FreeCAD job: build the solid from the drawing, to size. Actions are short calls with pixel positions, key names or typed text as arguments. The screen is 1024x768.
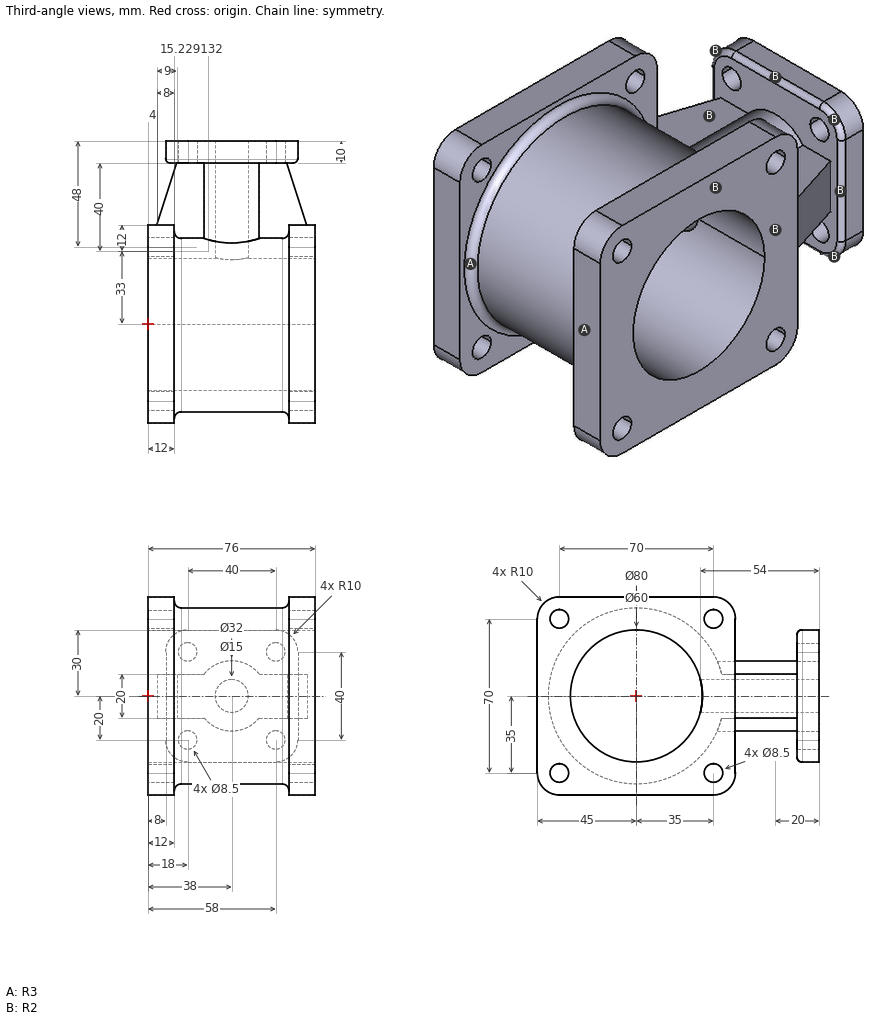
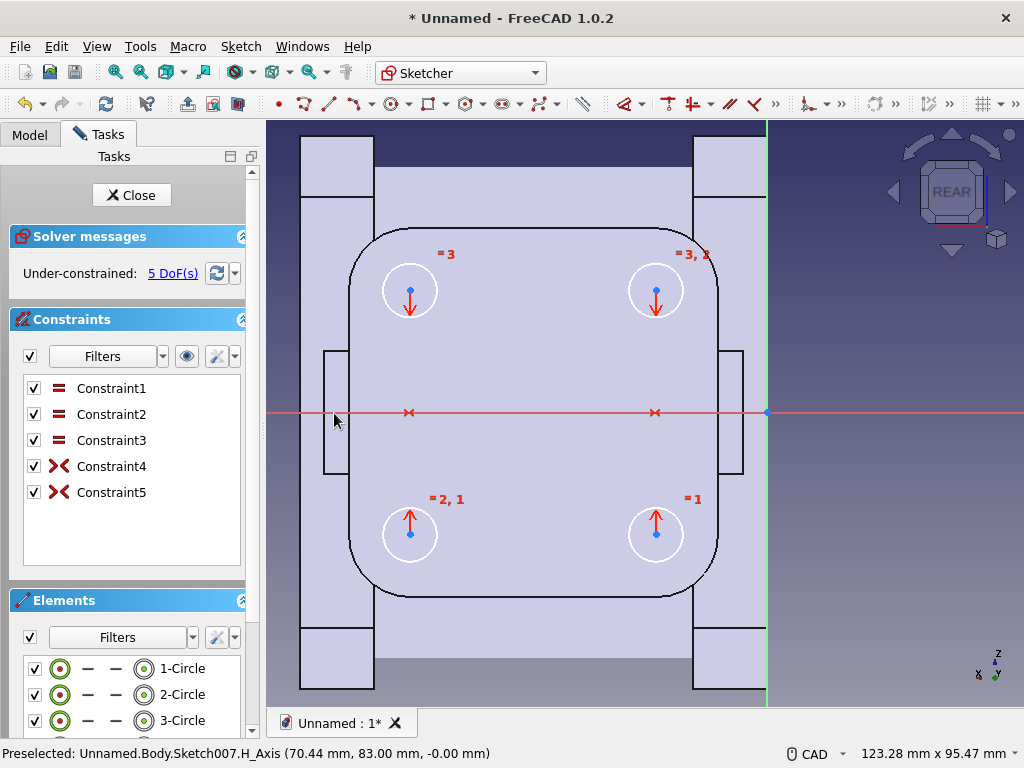
click(675, 516)
click(698, 493)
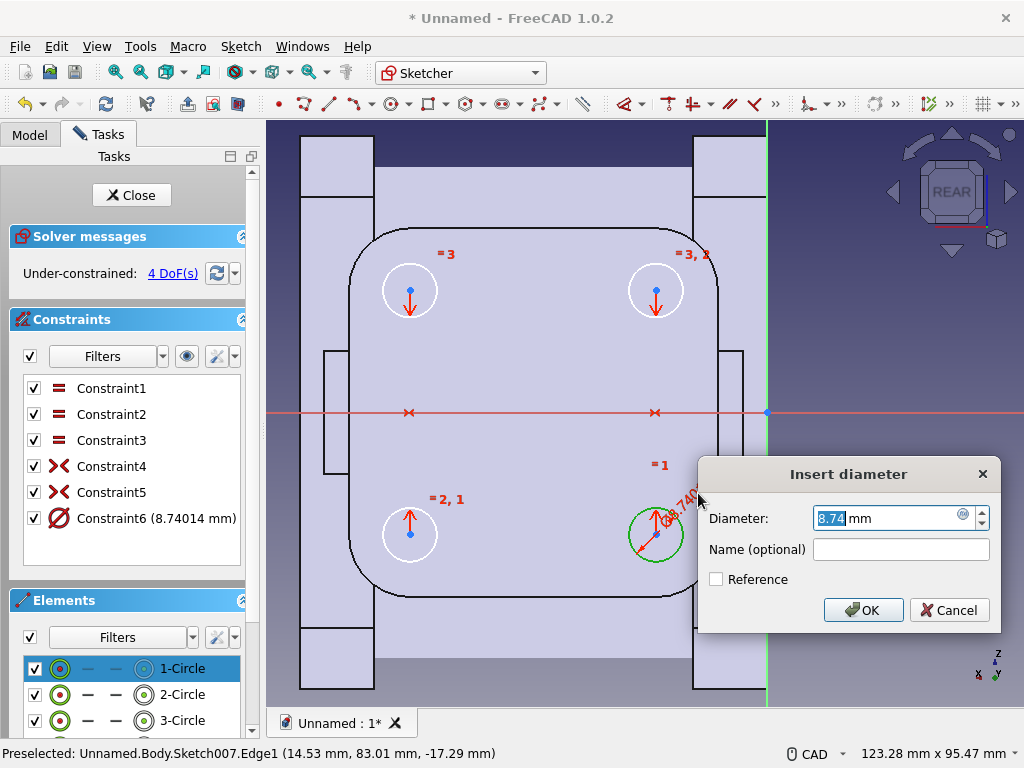
text(8.5)
key(Return)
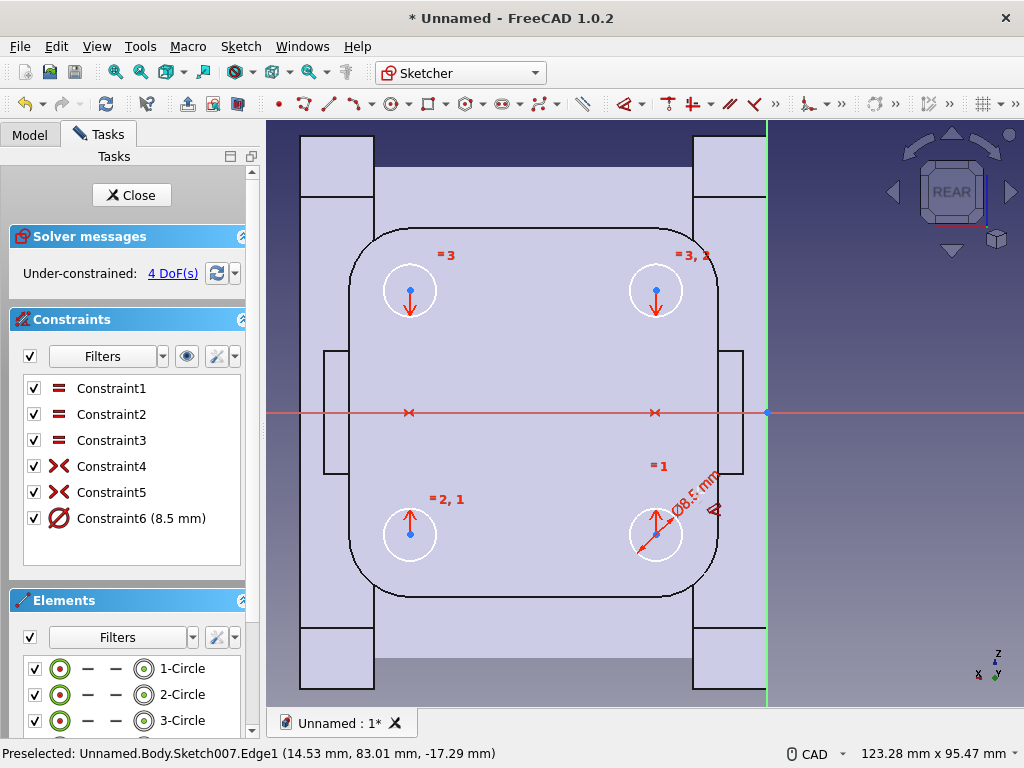
click(656, 535)
click(712, 569)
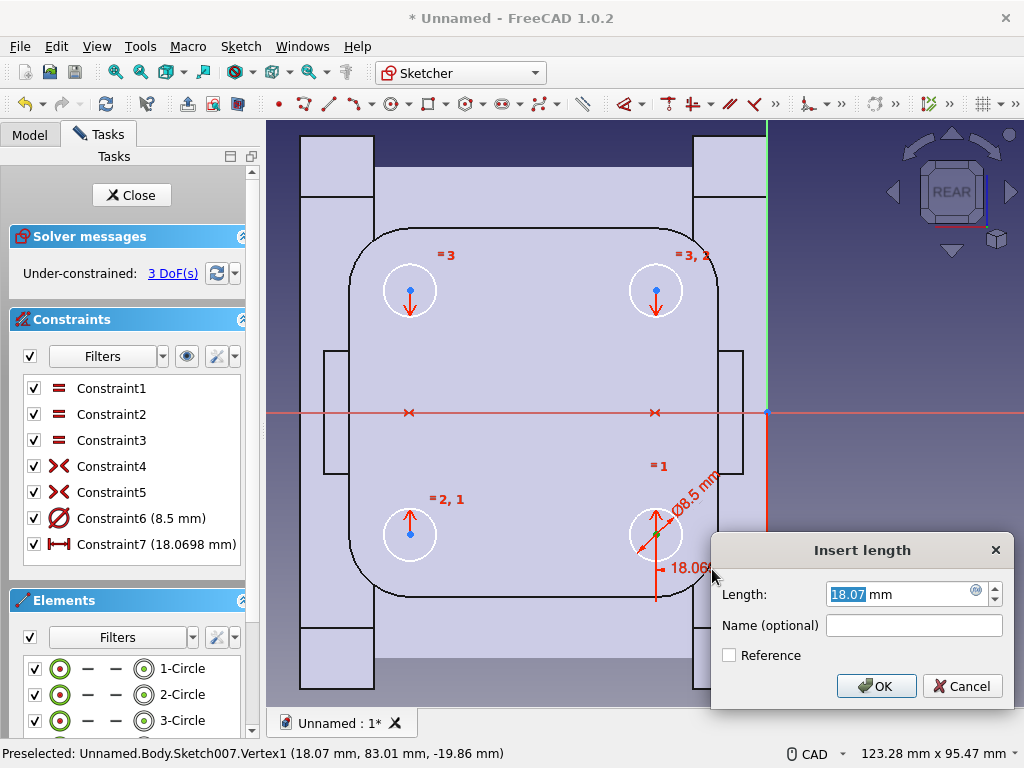
text(18)
key(Return)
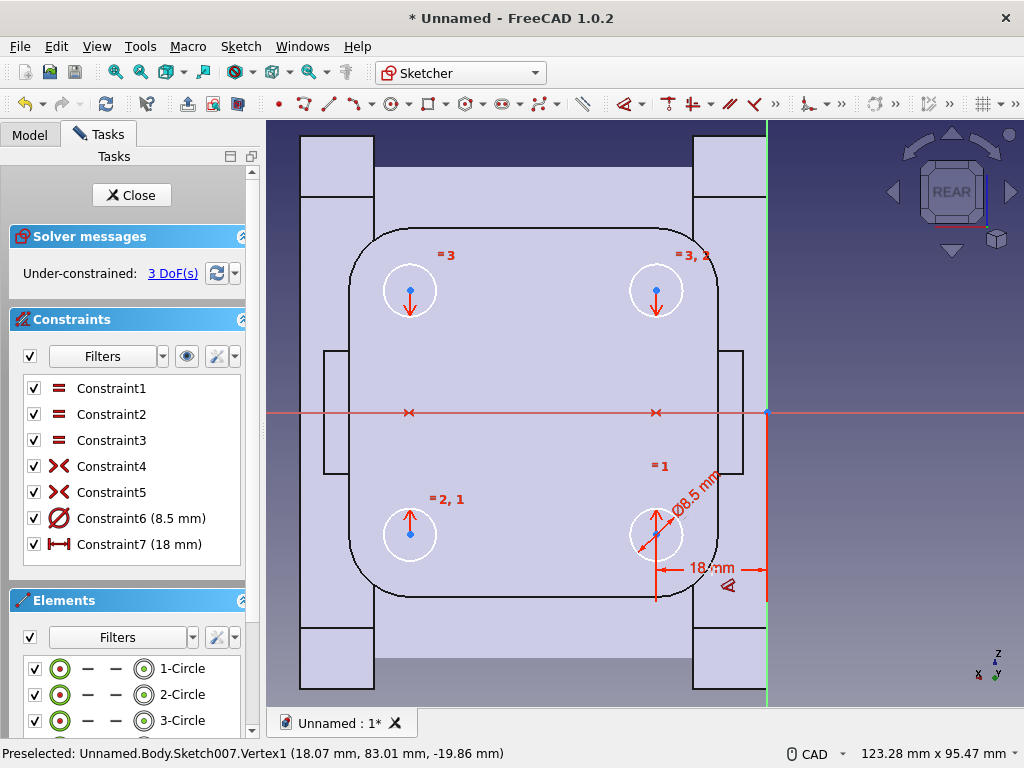
click(656, 535)
click(801, 474)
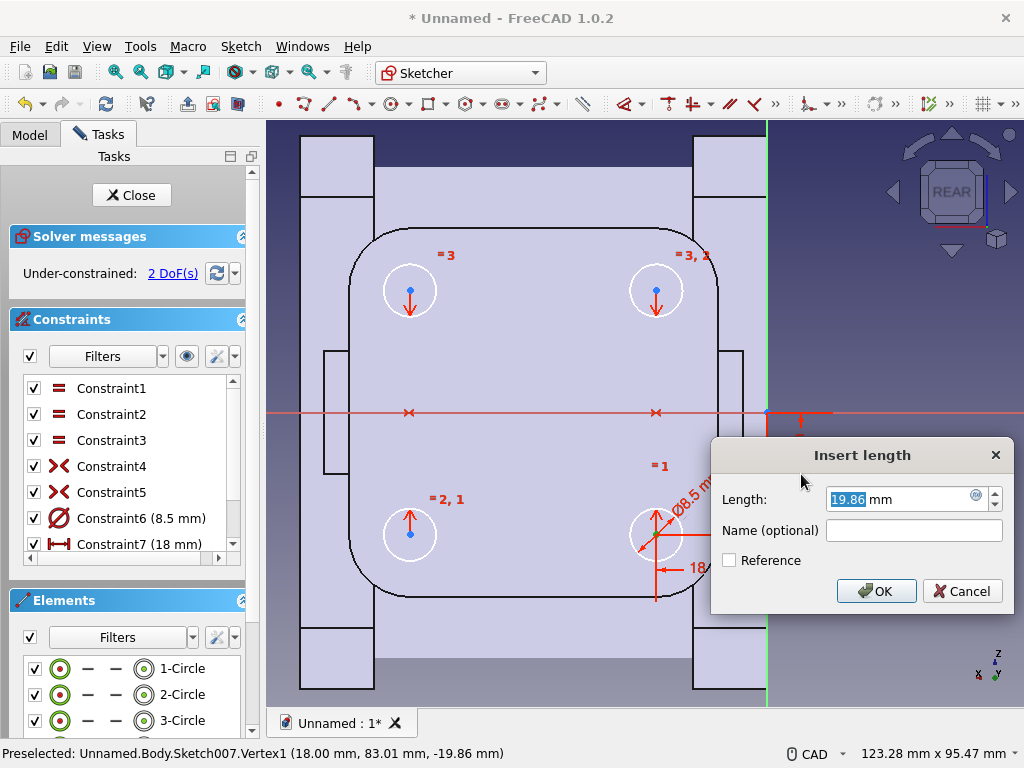
text(20)
key(Return)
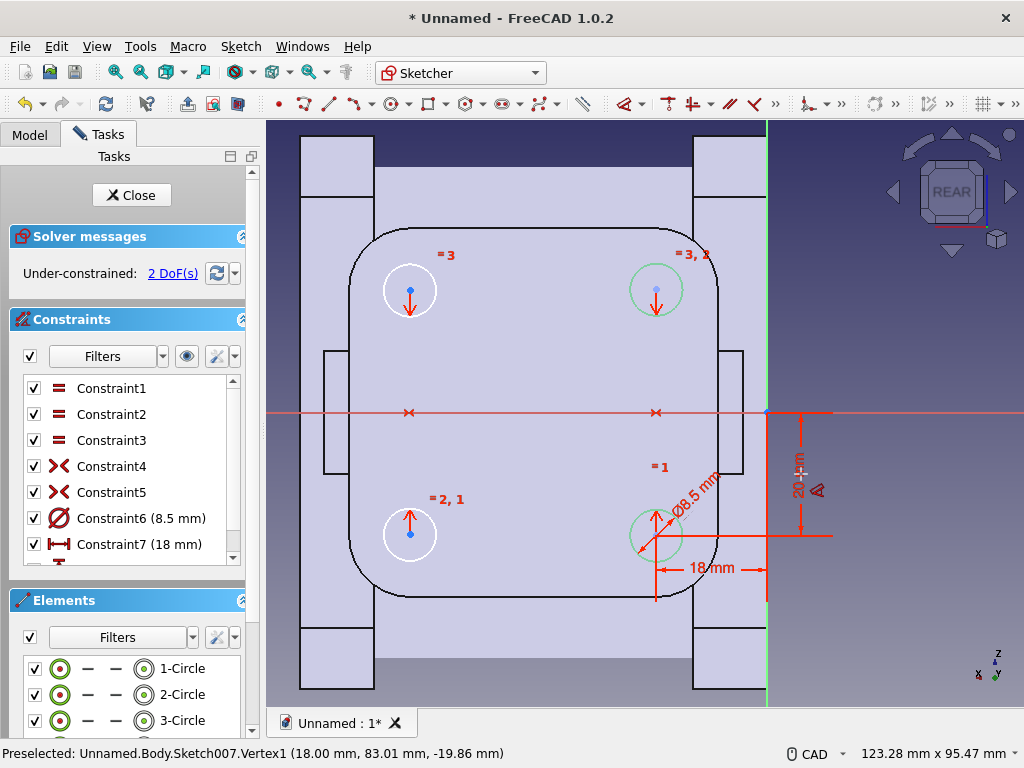
click(410, 535)
click(589, 569)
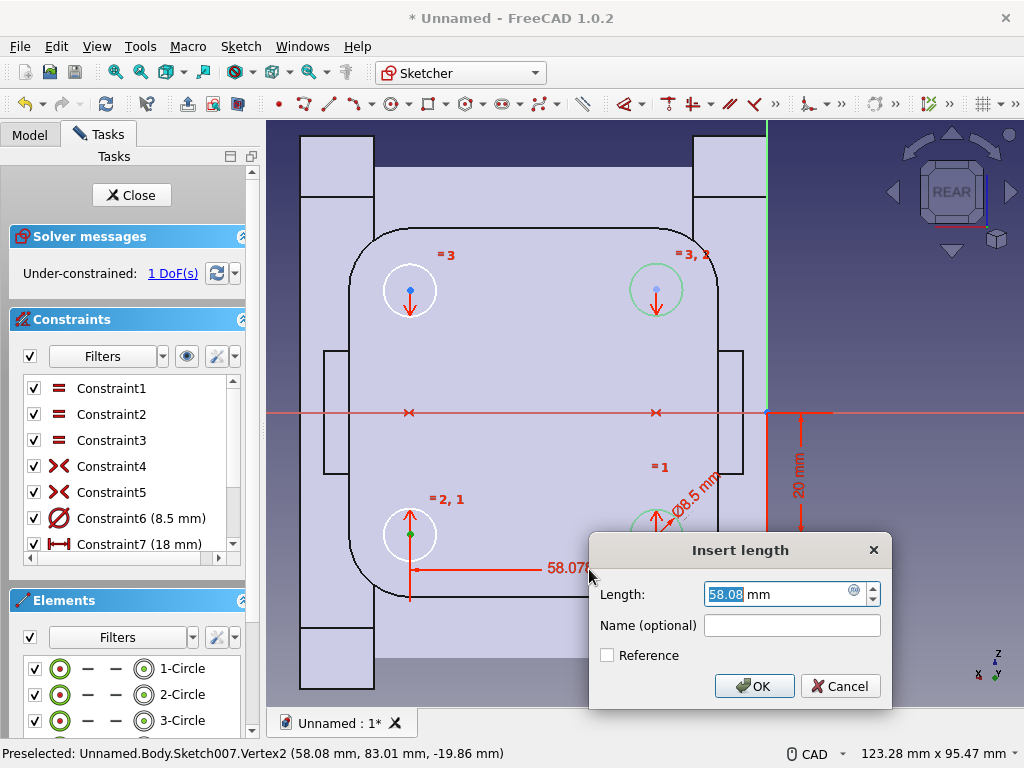
text(58)
key(Return)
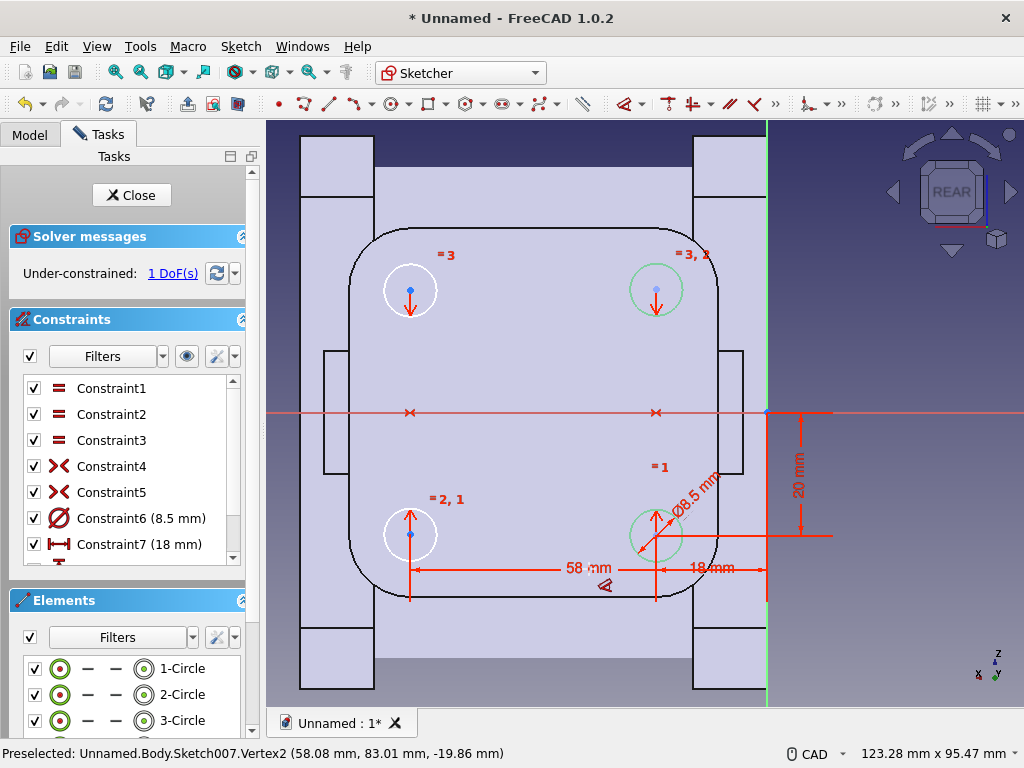
click(410, 535)
click(801, 446)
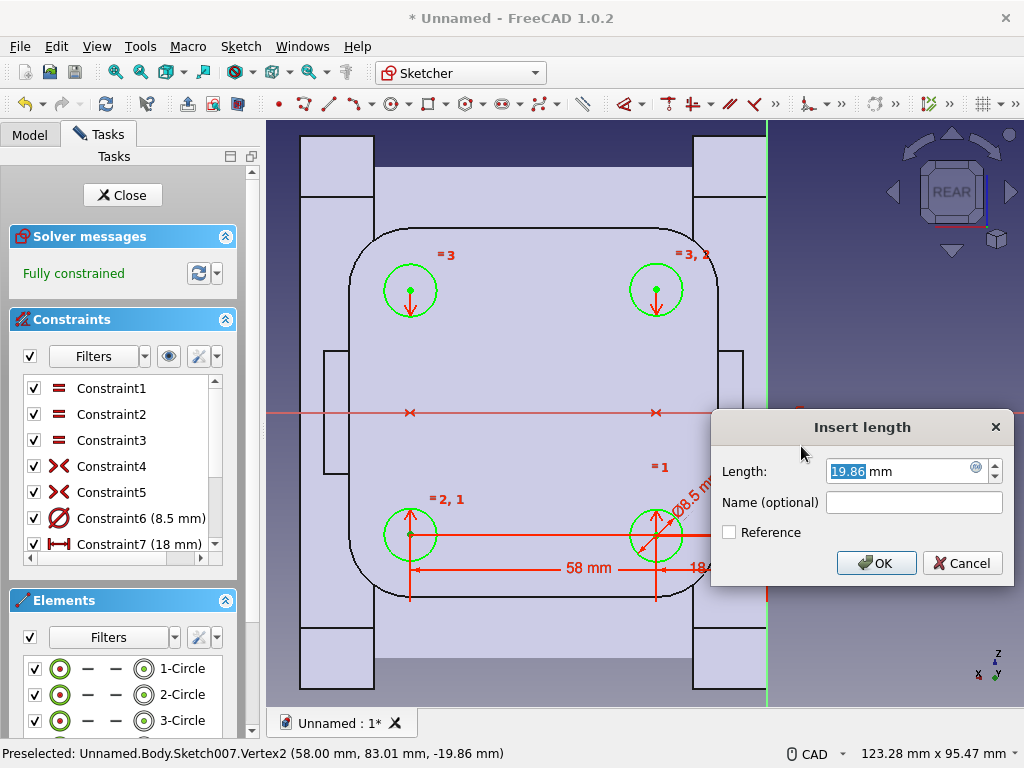
text(20)
key(Return)
key(Escape)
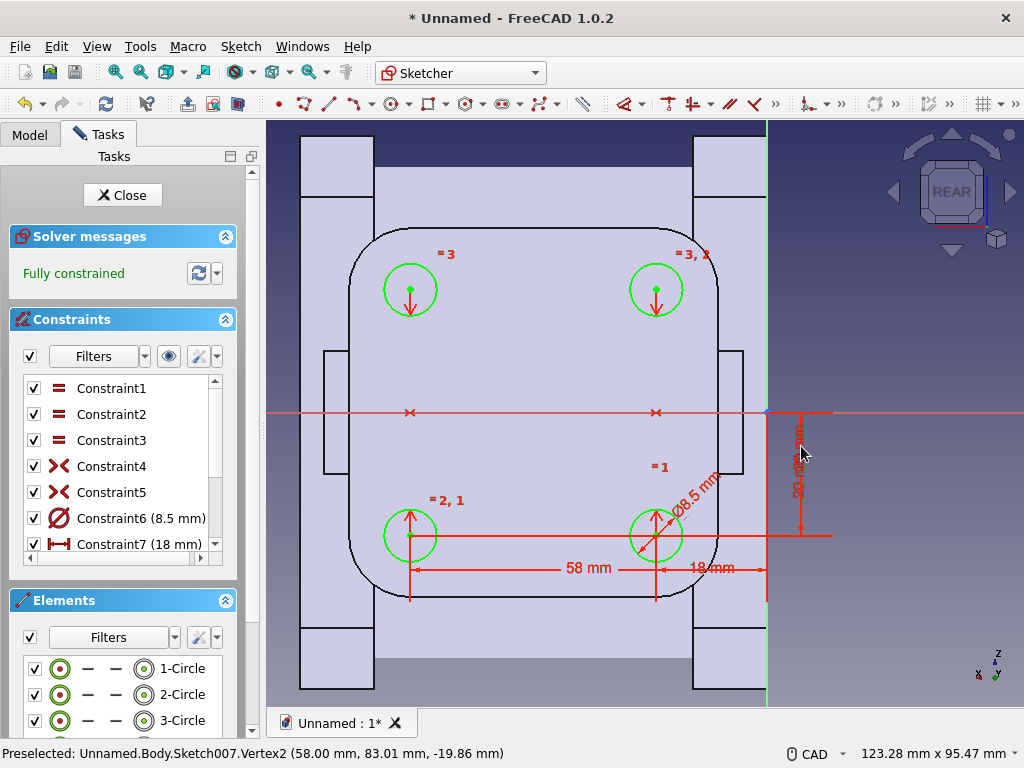
click(123, 195)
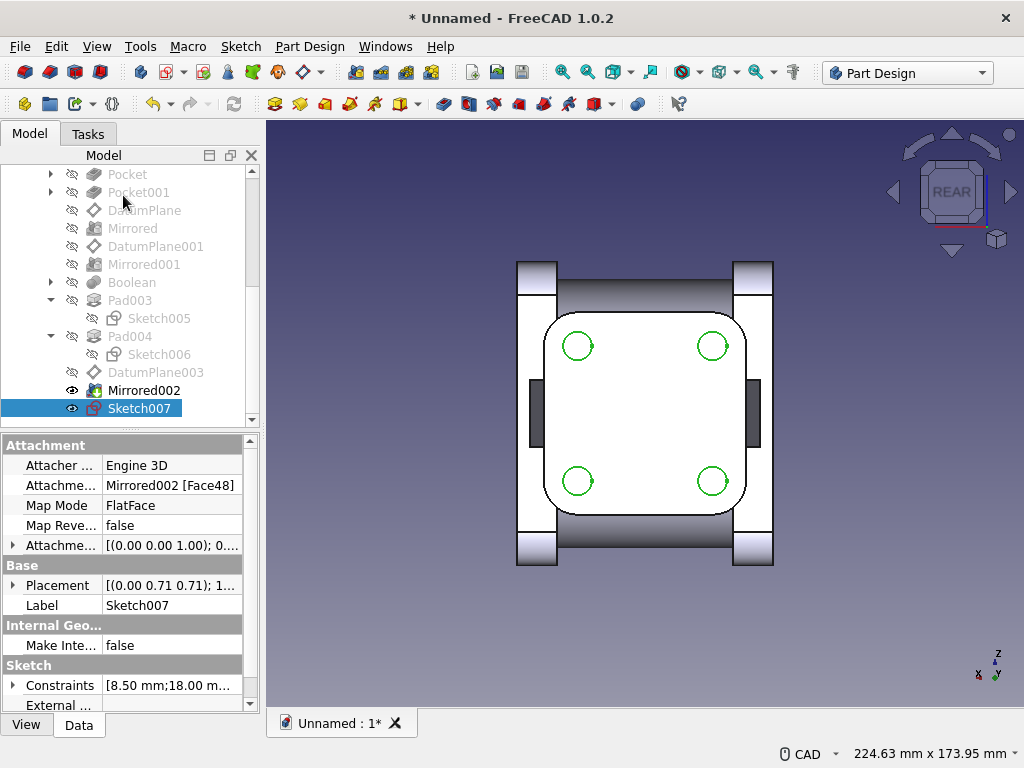
click(444, 104)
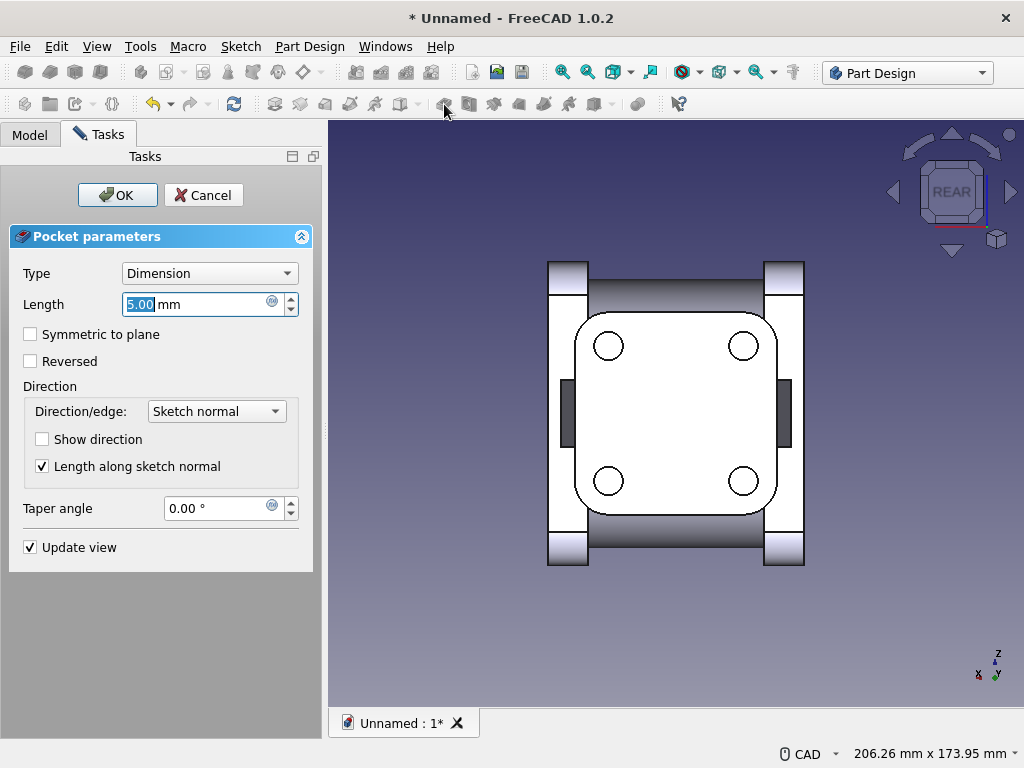
text(20)
key(Tab)